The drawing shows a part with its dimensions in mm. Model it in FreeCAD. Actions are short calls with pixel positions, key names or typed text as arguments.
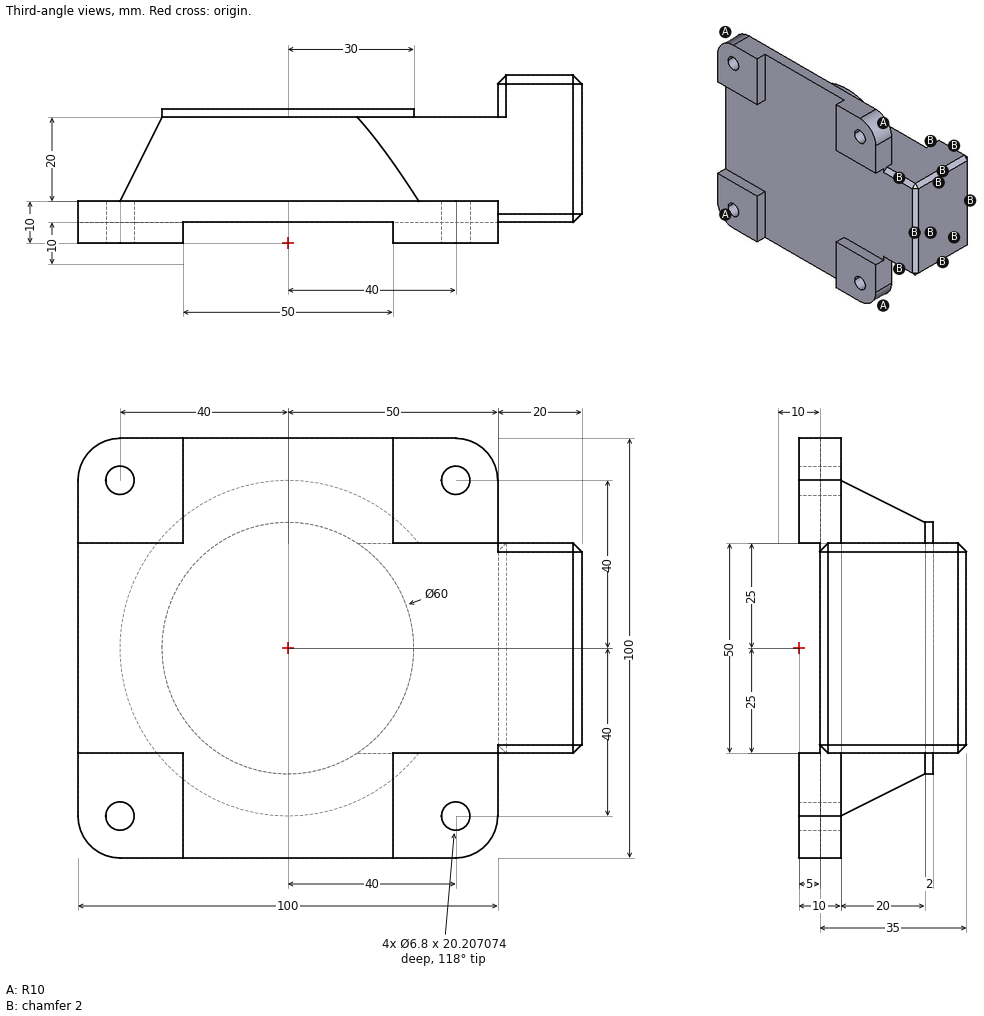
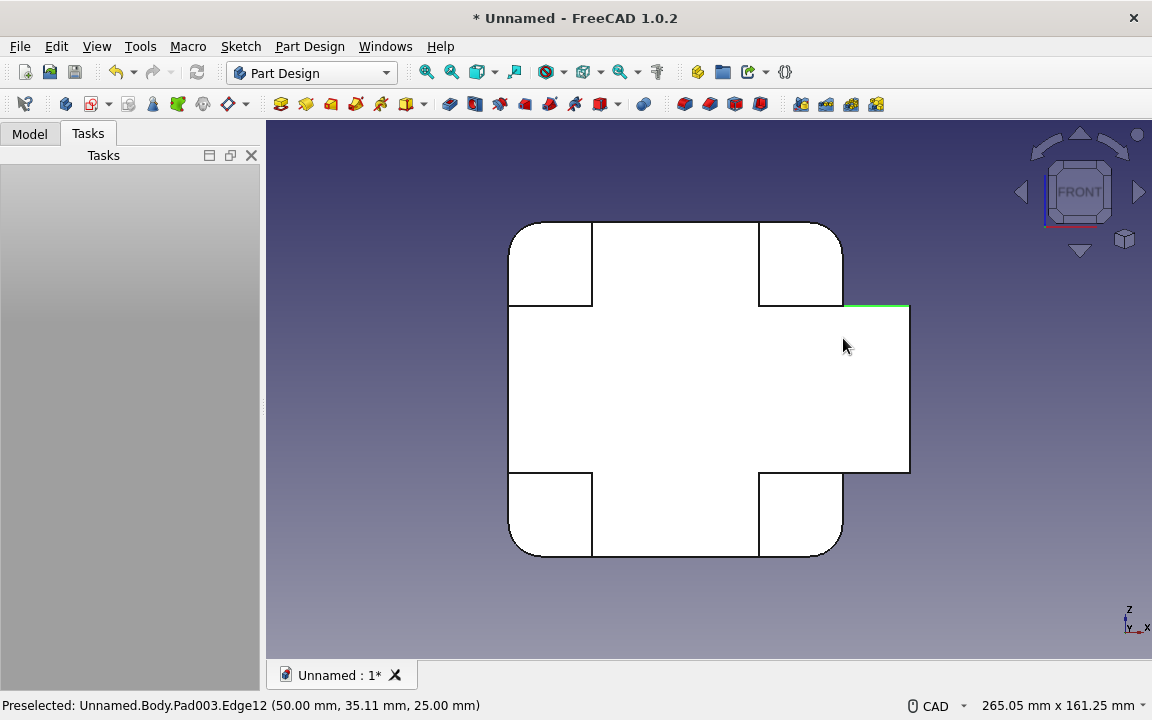
key(3)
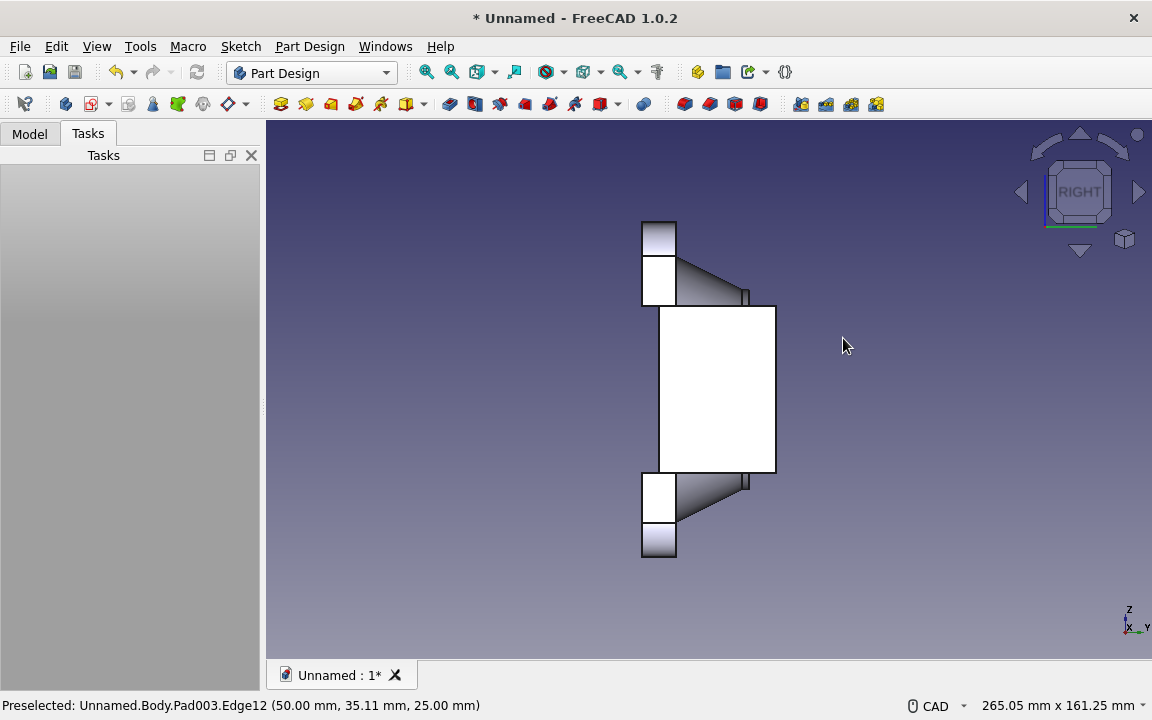
key(5)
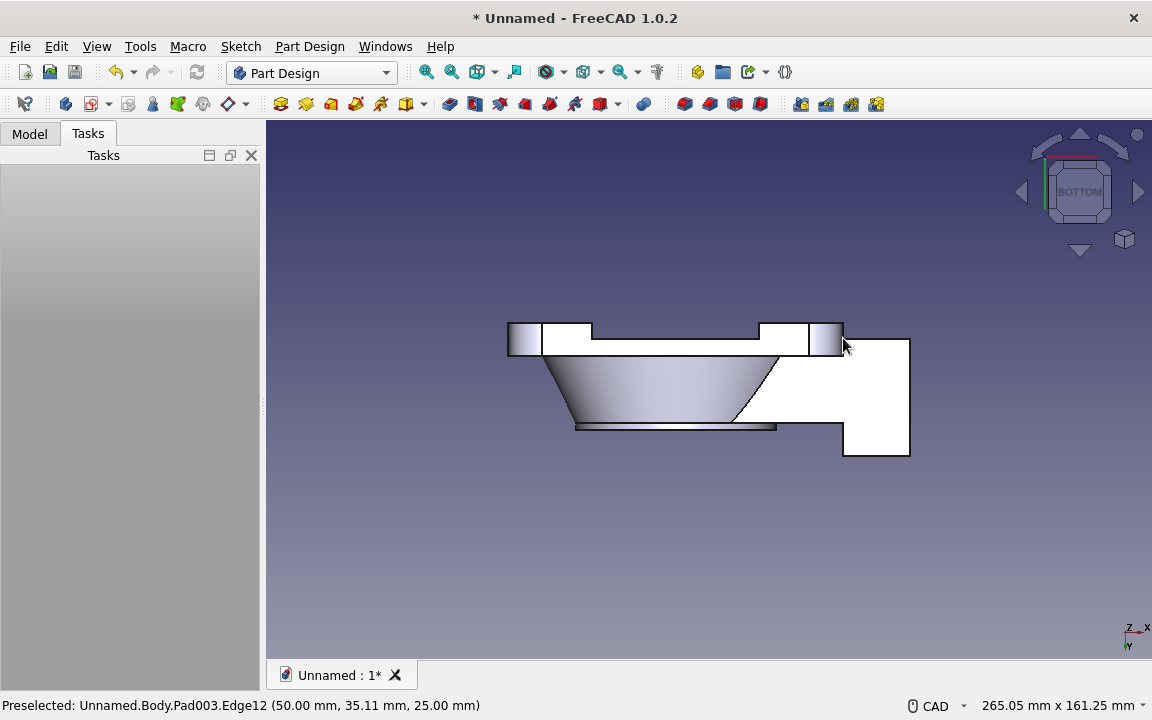
click(876, 338, ctrl)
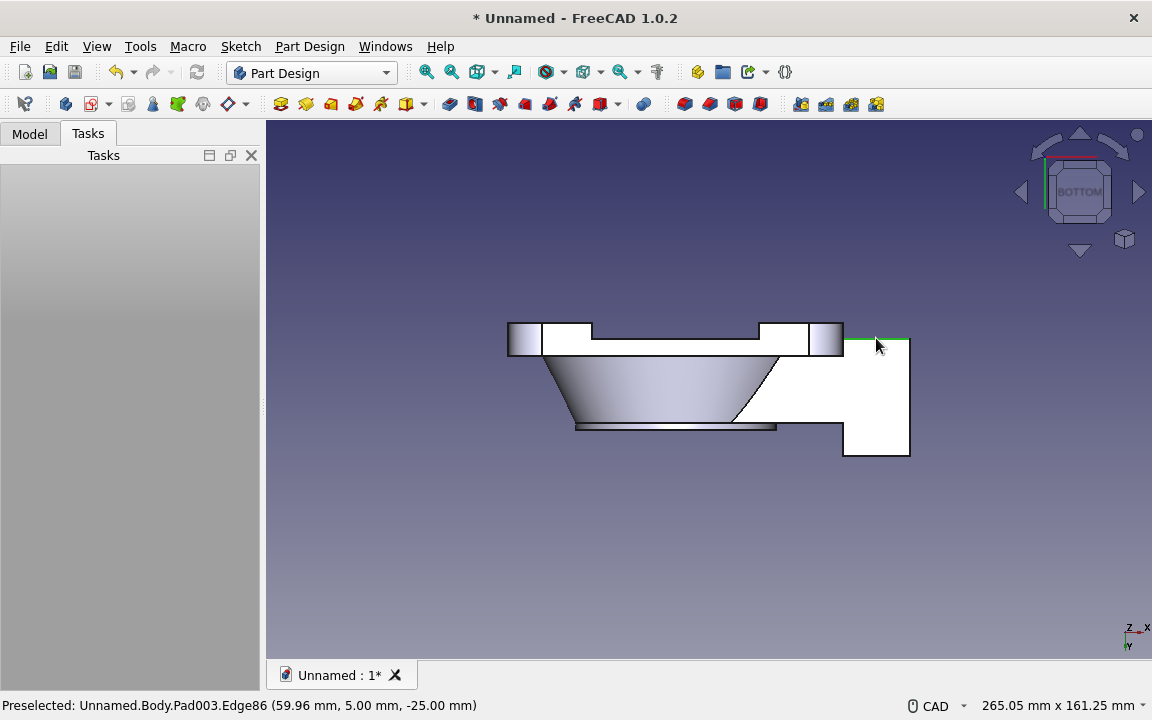
click(843, 439, ctrl)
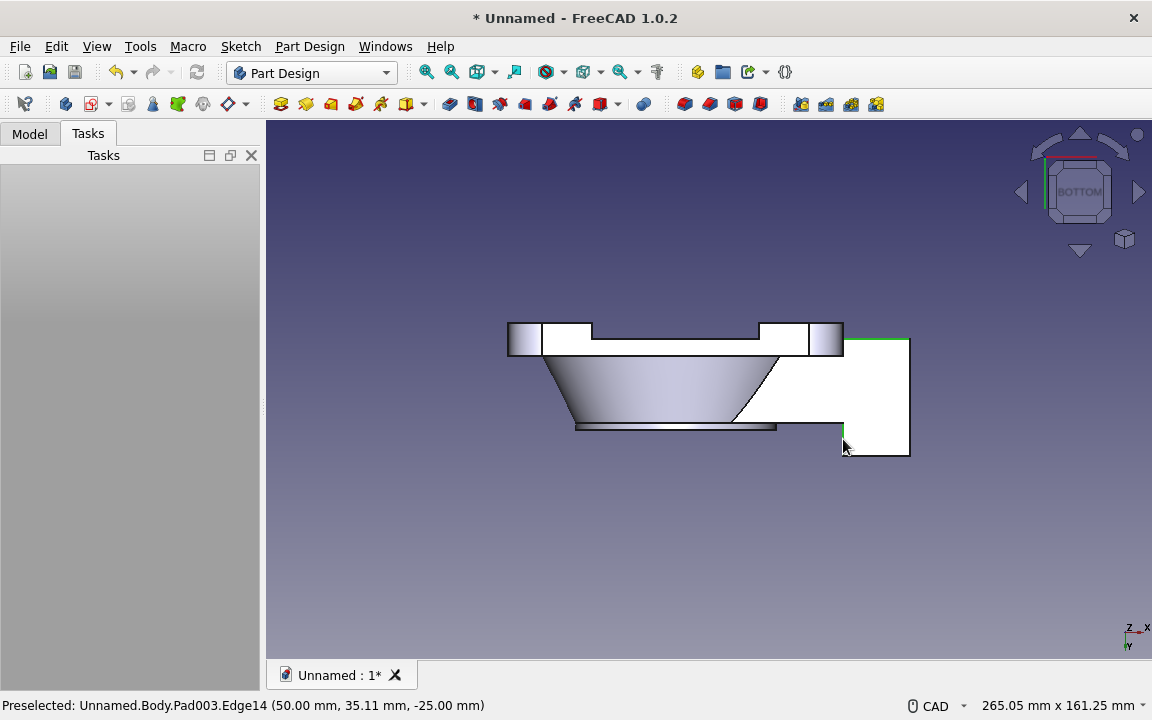
key(4)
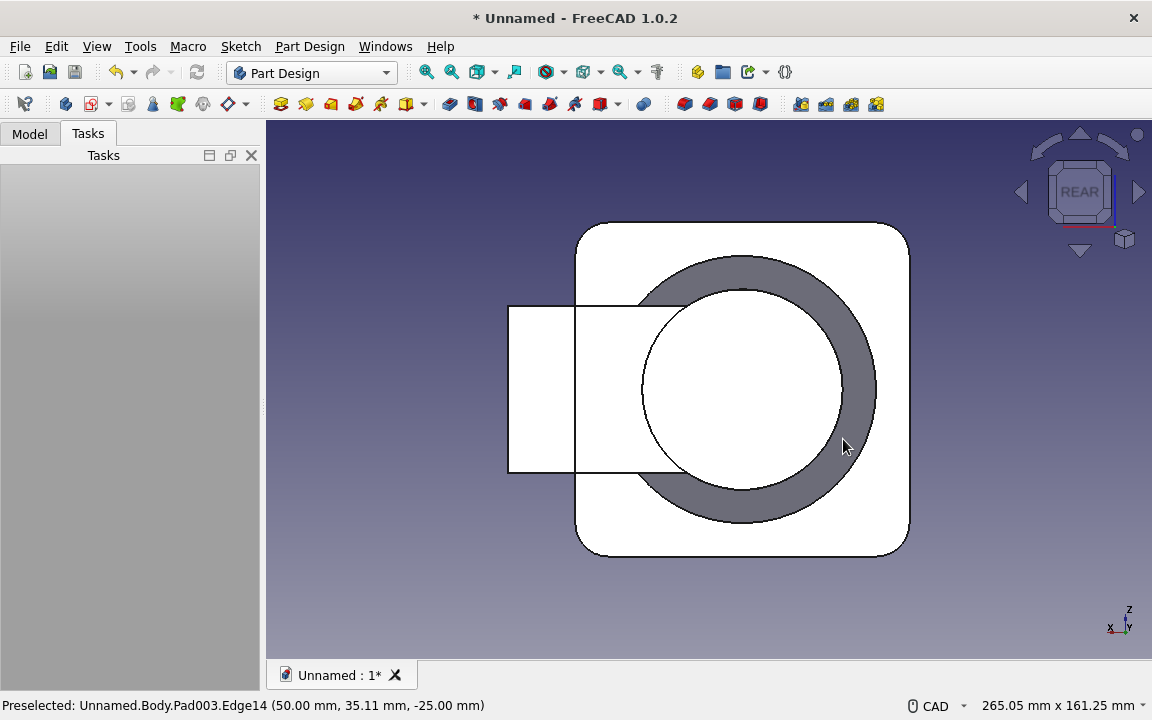
click(542, 341, ctrl)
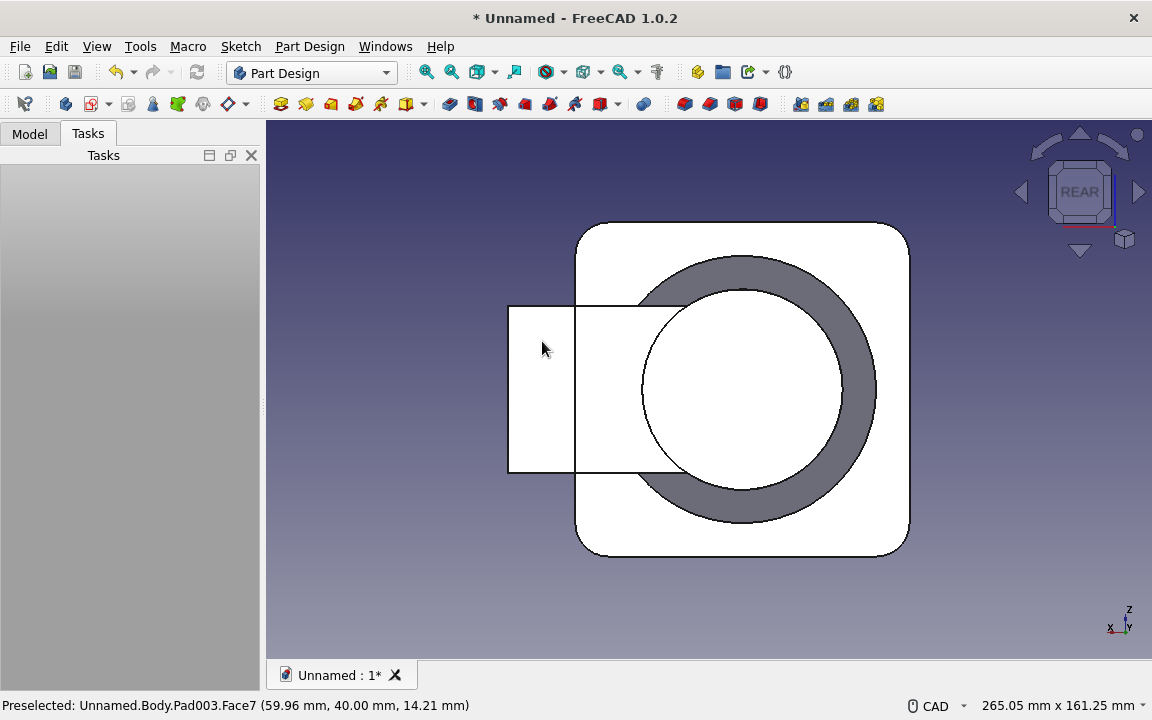
click(710, 104)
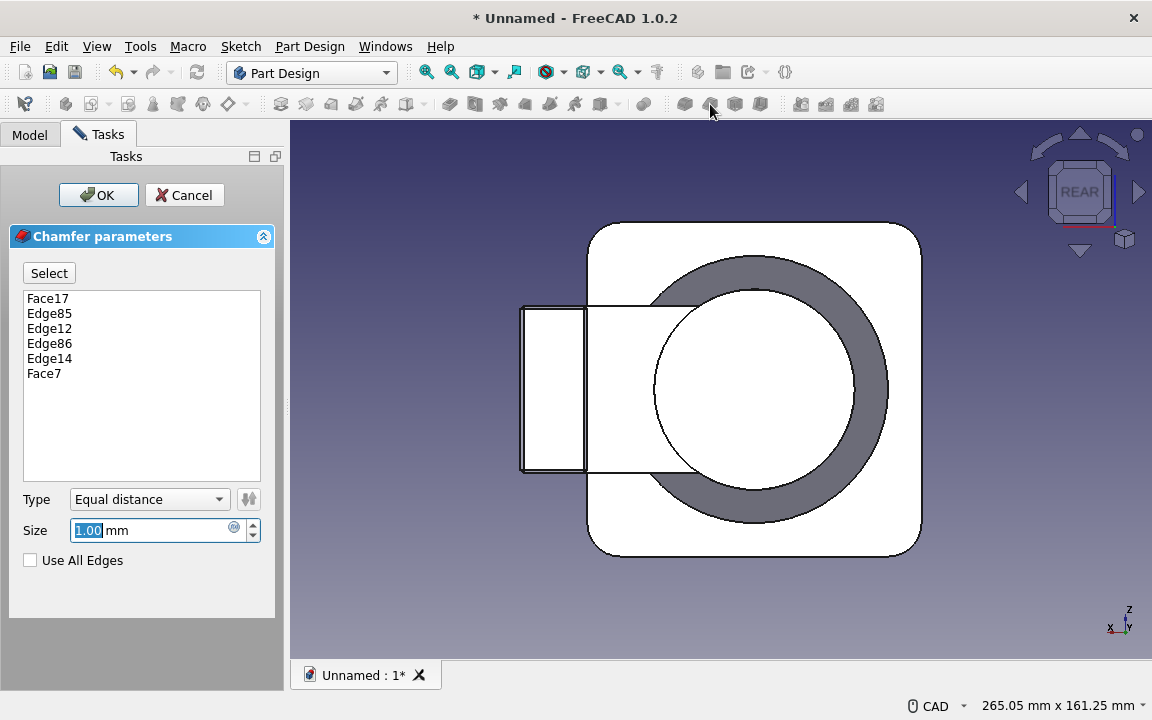
text(2)
key(Tab)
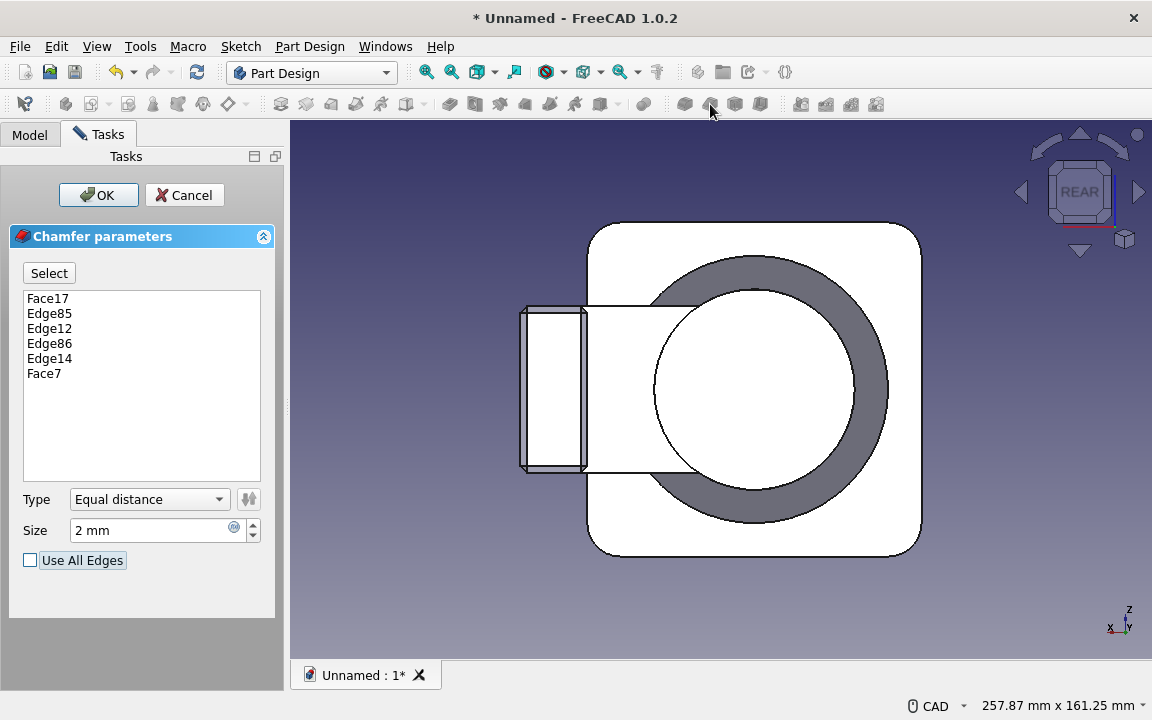
click(99, 195)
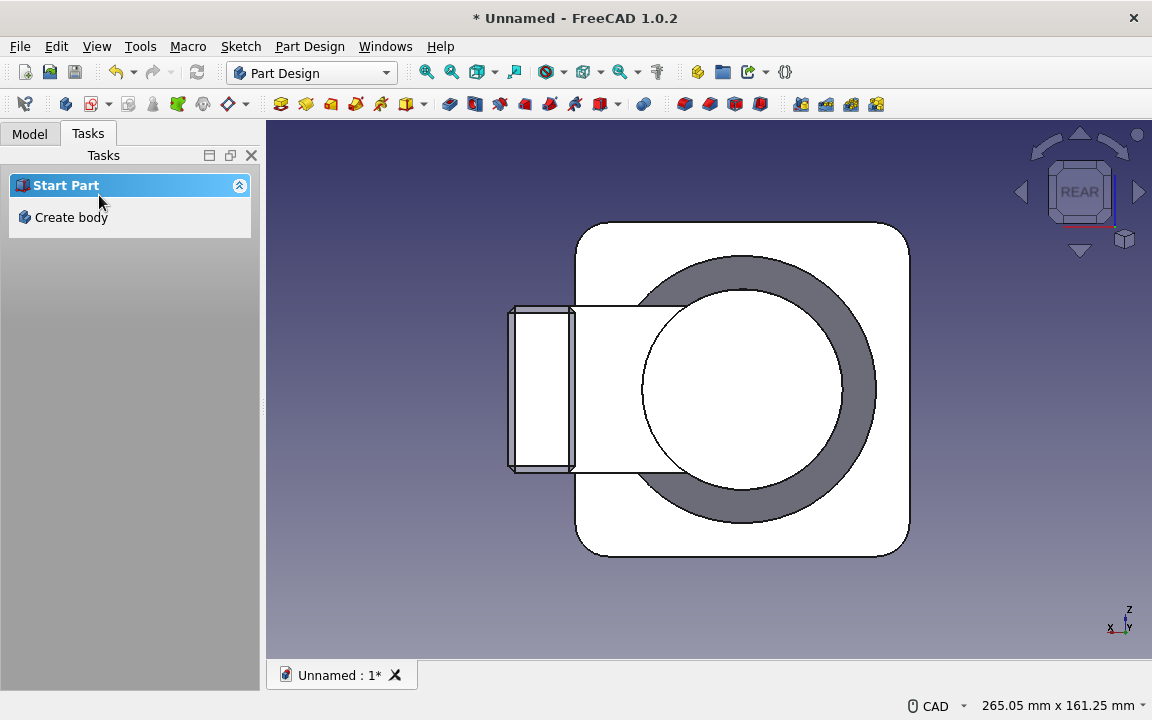
click(647, 245)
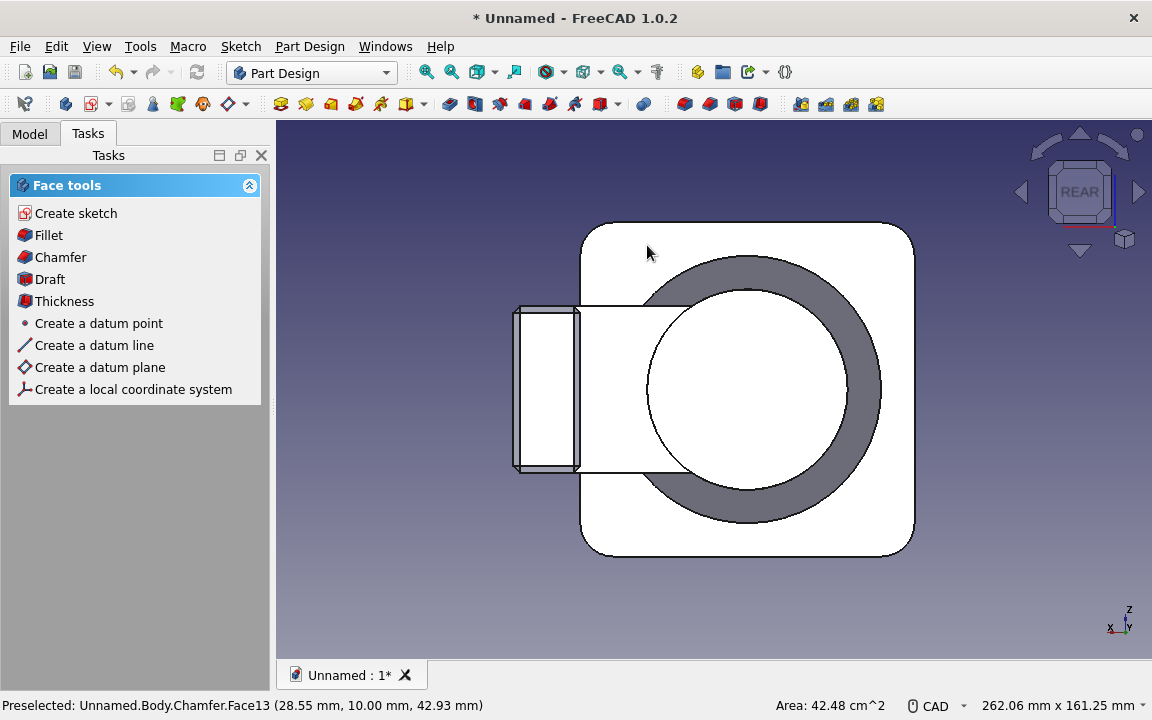
click(90, 104)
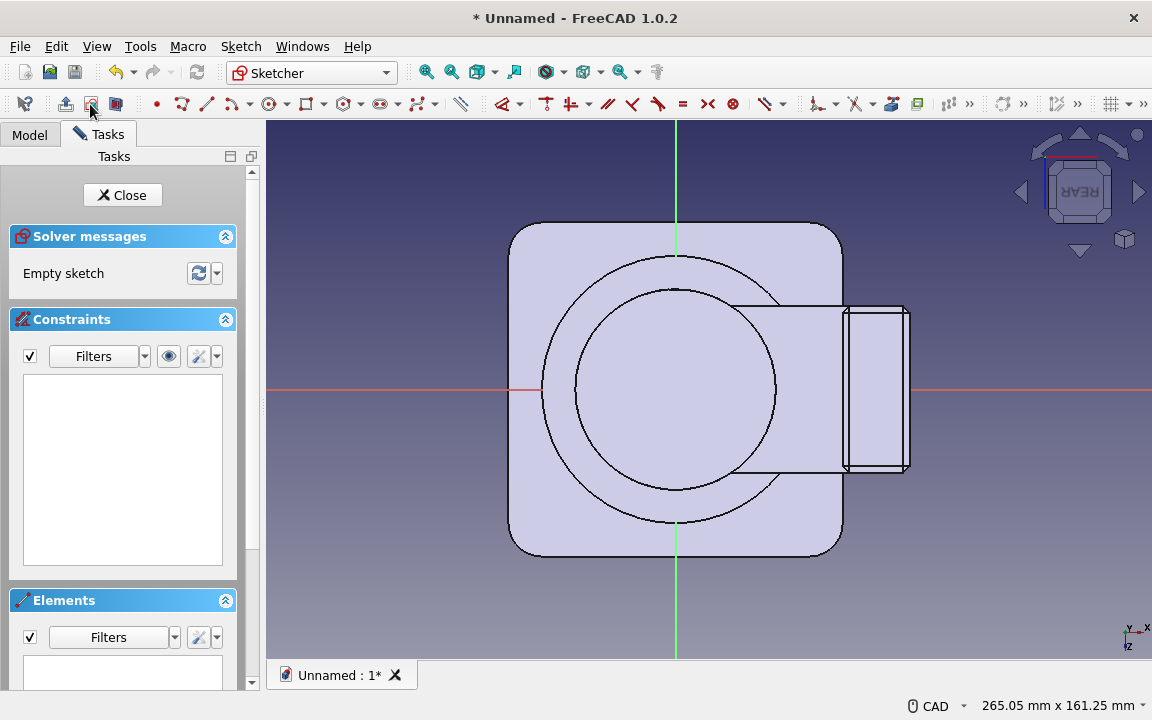
key(g)
key(c)